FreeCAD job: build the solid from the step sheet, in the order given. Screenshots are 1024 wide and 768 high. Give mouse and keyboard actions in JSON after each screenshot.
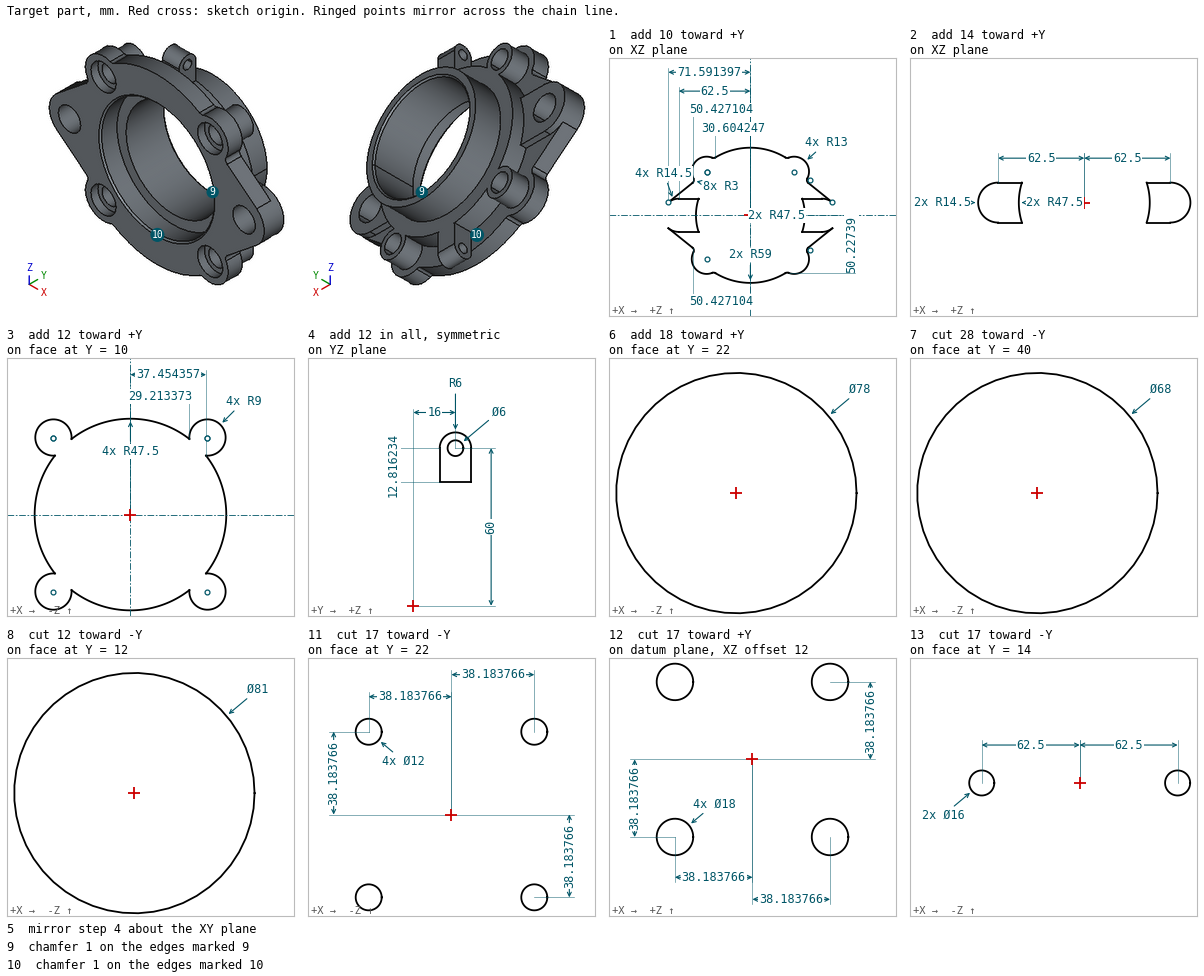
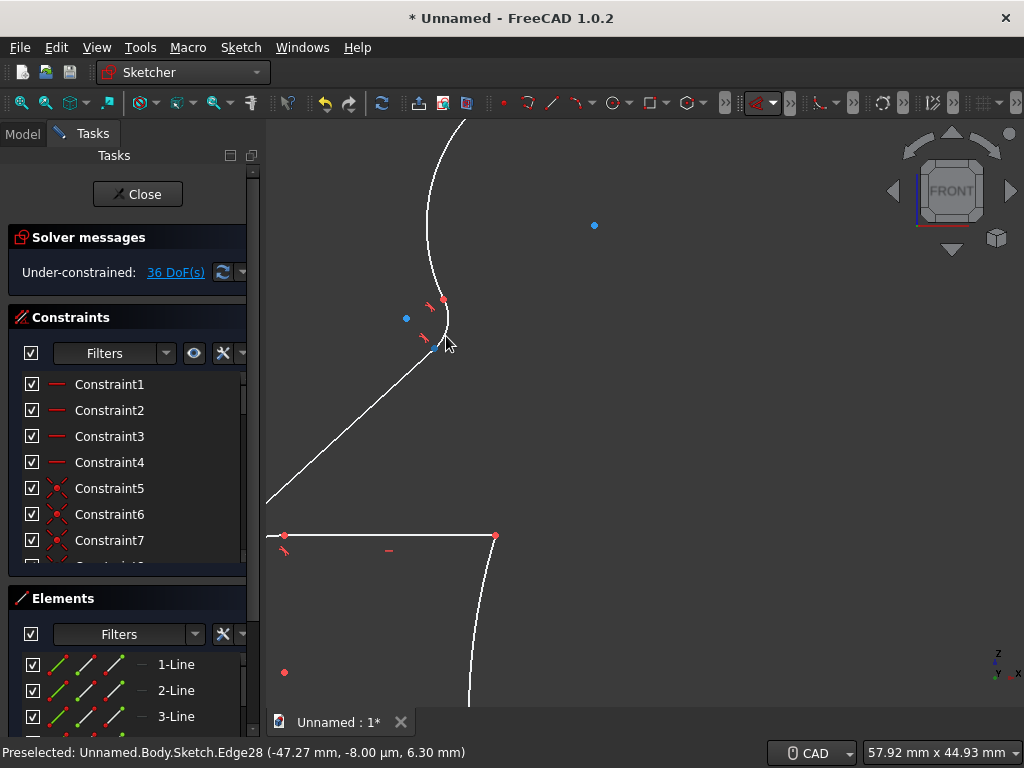
{"action": "left_click", "coordinate": [444, 336]}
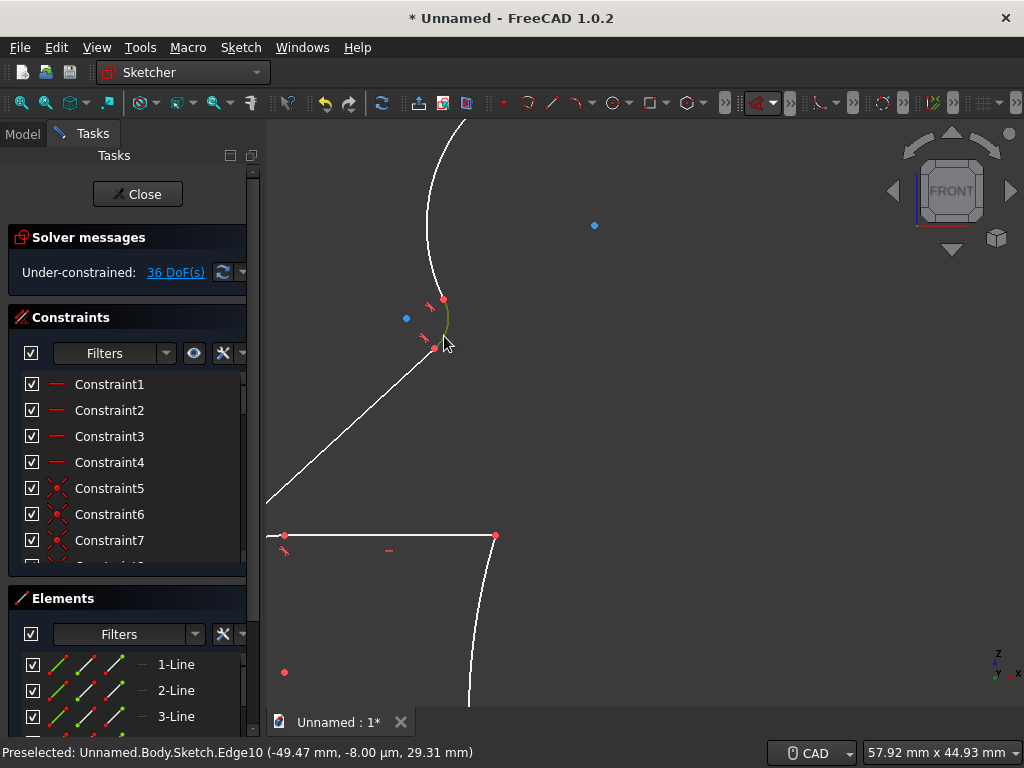
{"action": "scroll", "coordinate": [446, 336], "scroll_direction": "down", "scroll_amount": 8}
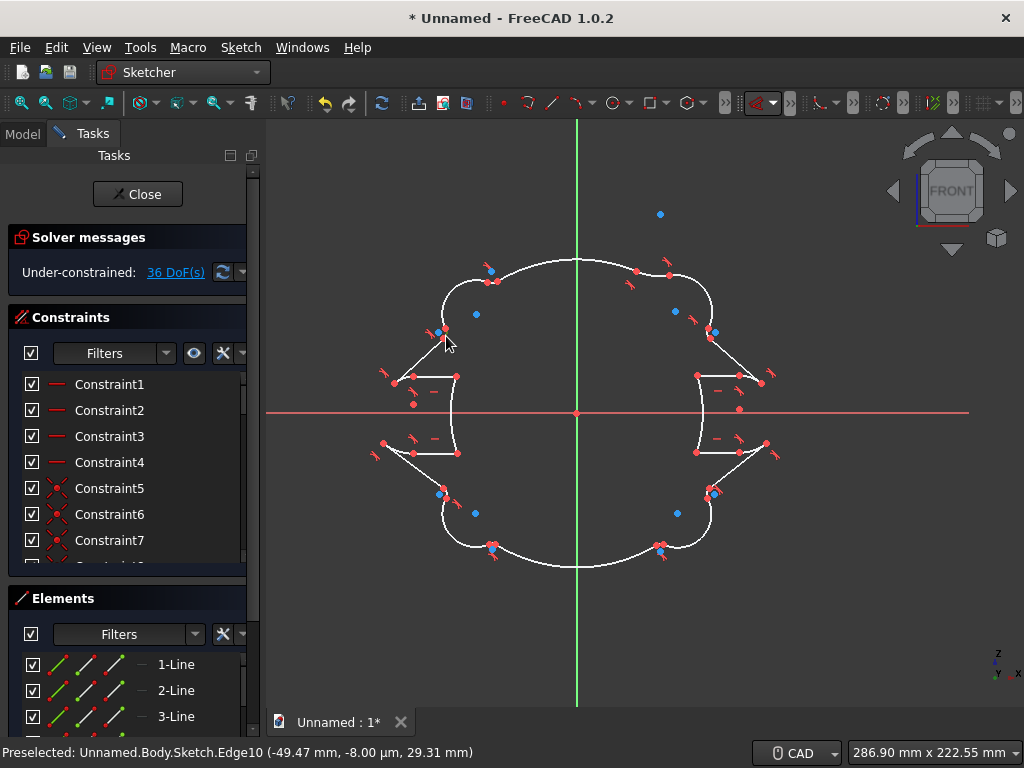
{"action": "scroll", "coordinate": [491, 283], "scroll_direction": "up", "scroll_amount": 8}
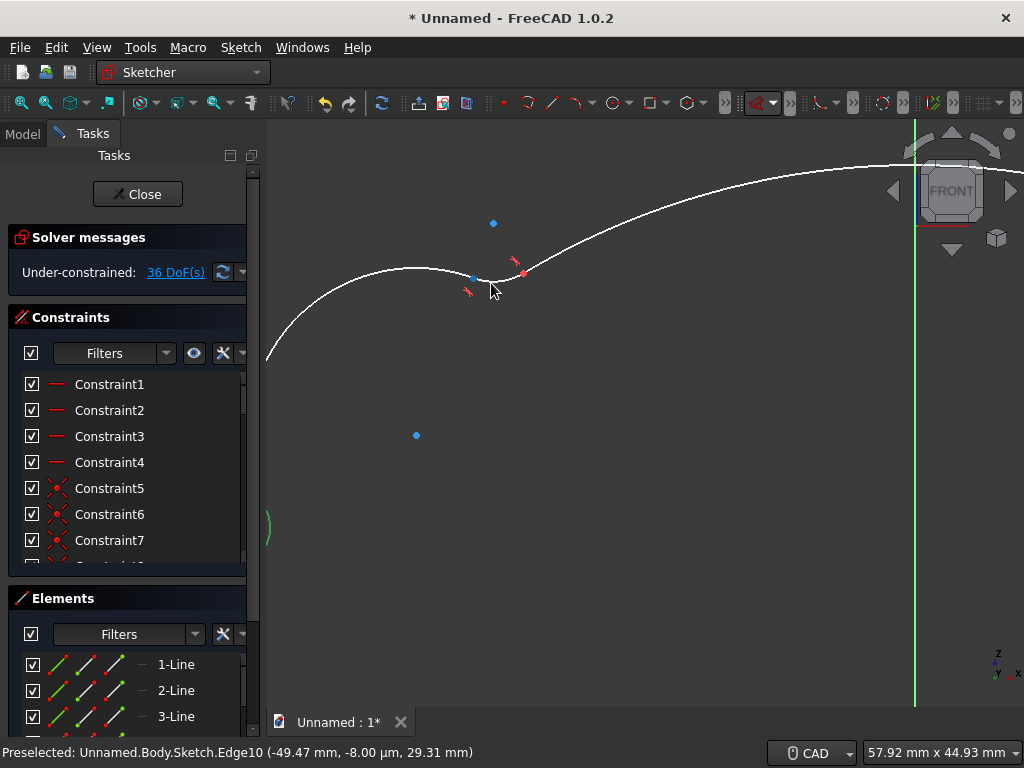
{"action": "left_click", "coordinate": [489, 281]}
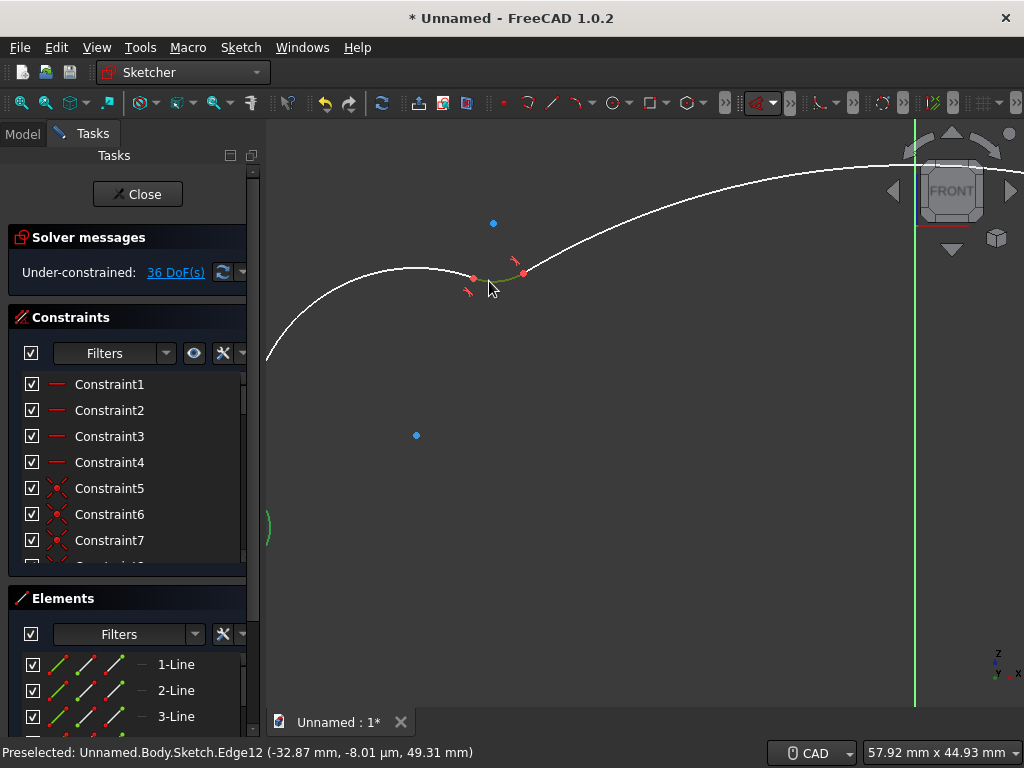
{"action": "scroll", "coordinate": [491, 283], "scroll_direction": "down", "scroll_amount": 8}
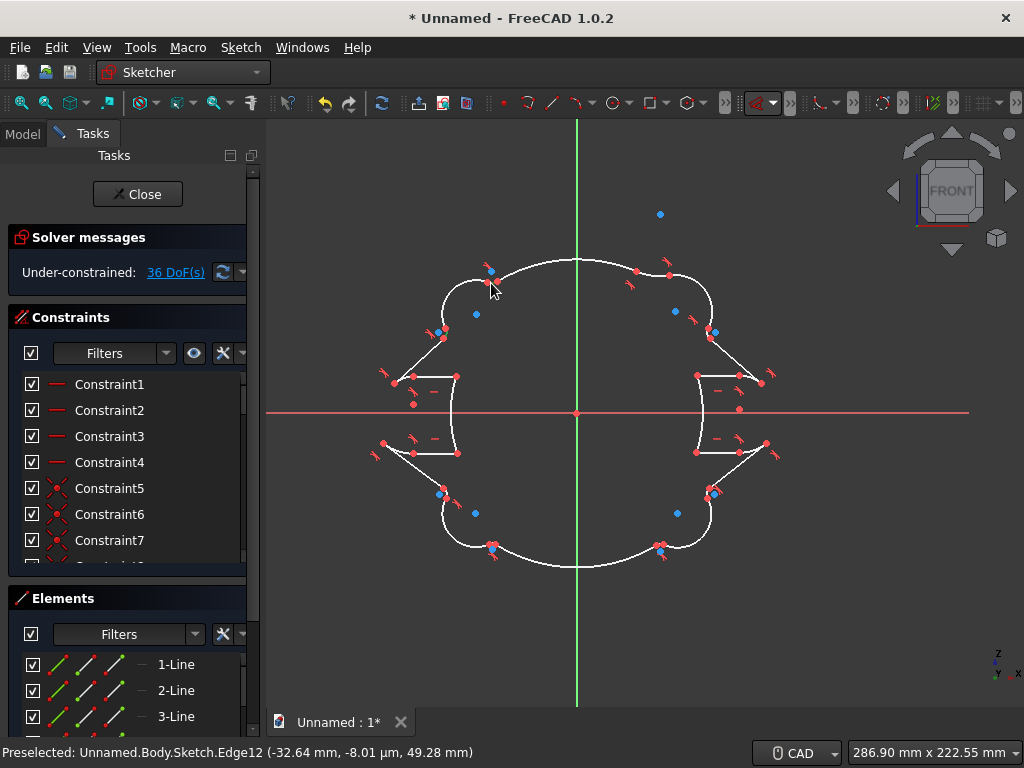
{"action": "scroll", "coordinate": [646, 275], "scroll_direction": "up", "scroll_amount": 2}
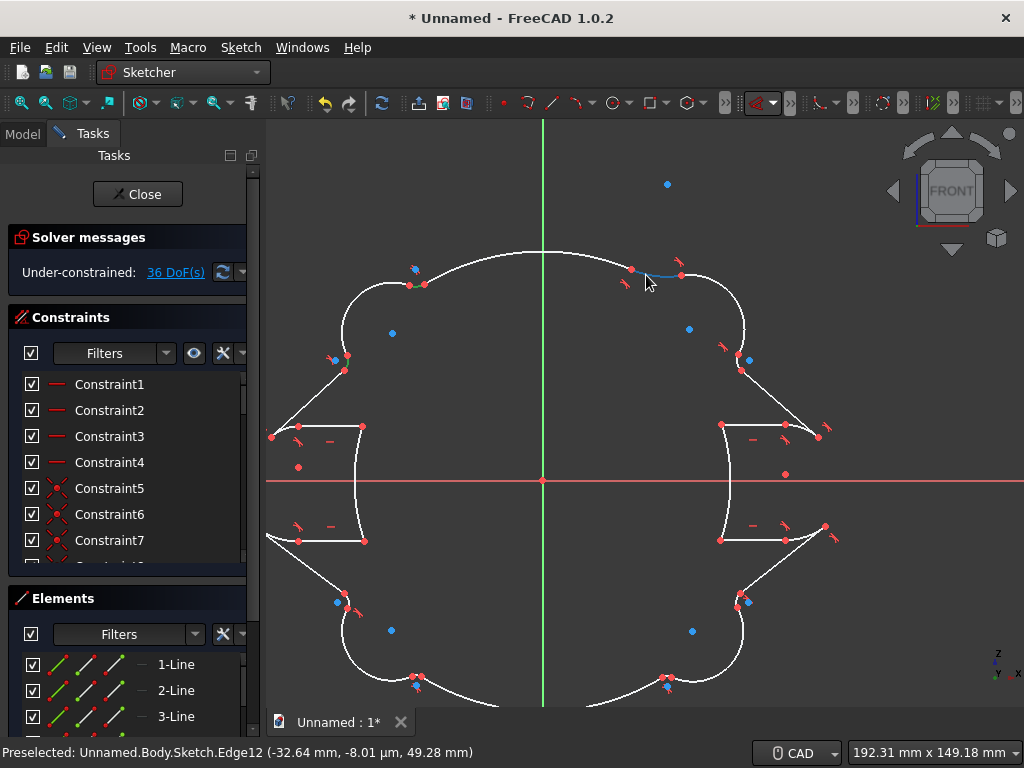
{"action": "left_click", "coordinate": [646, 274]}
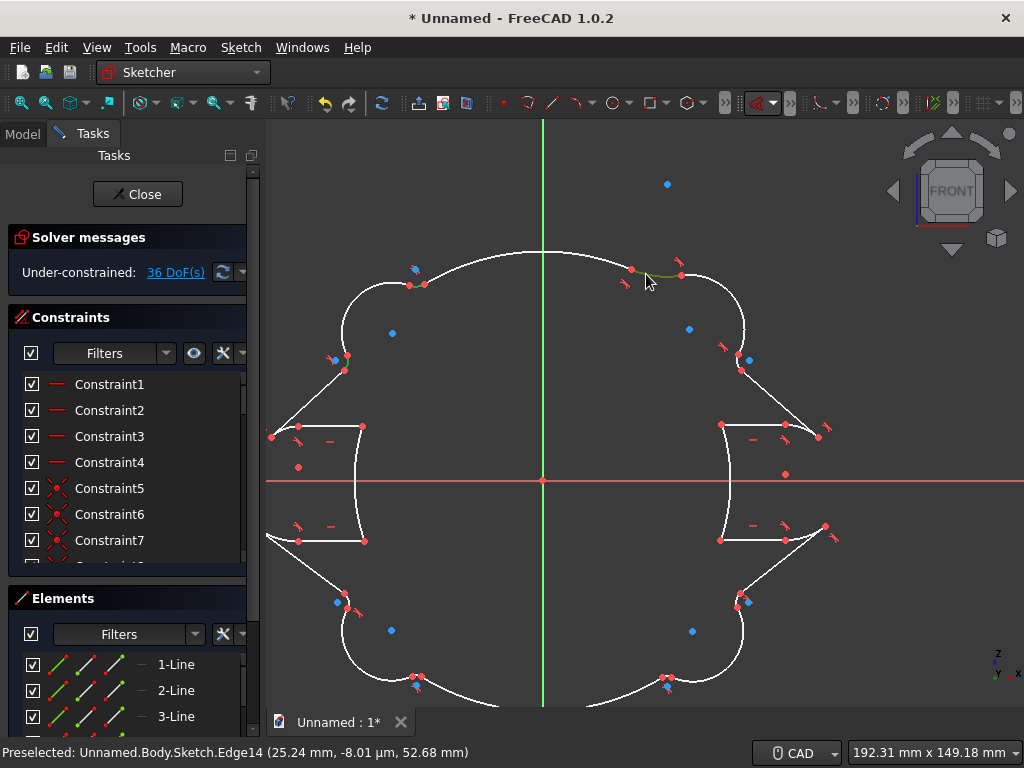
{"action": "scroll", "coordinate": [737, 363], "scroll_direction": "up", "scroll_amount": 3}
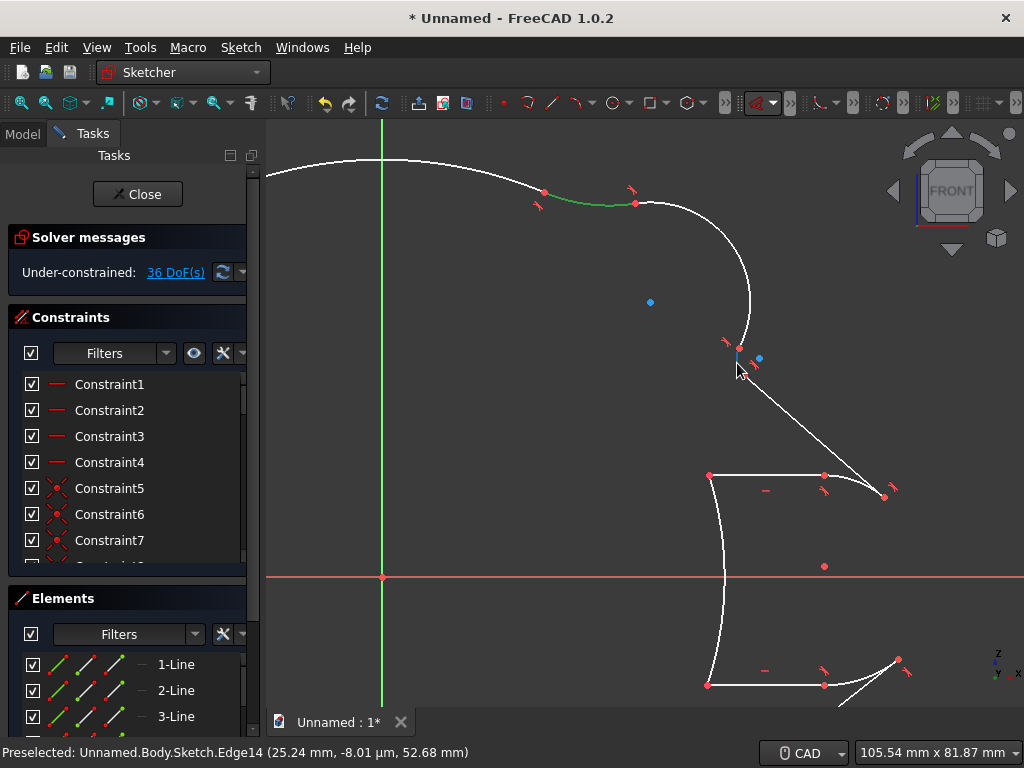
{"action": "left_click", "coordinate": [737, 363]}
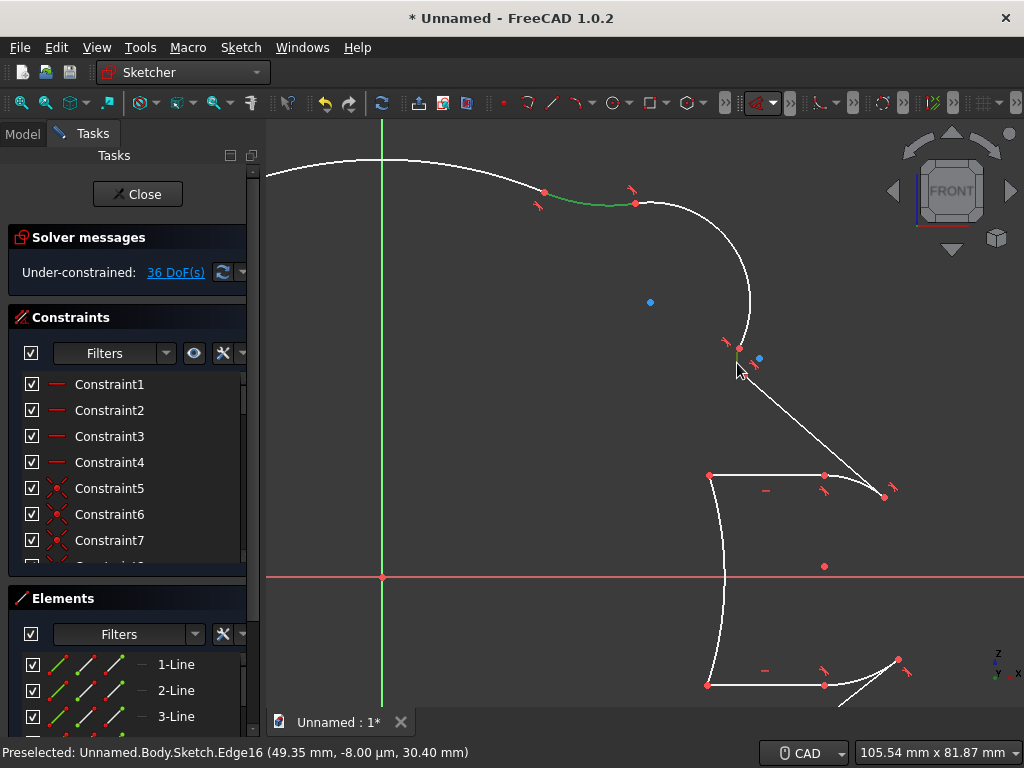
{"action": "scroll", "coordinate": [690, 317], "scroll_direction": "down", "scroll_amount": 5}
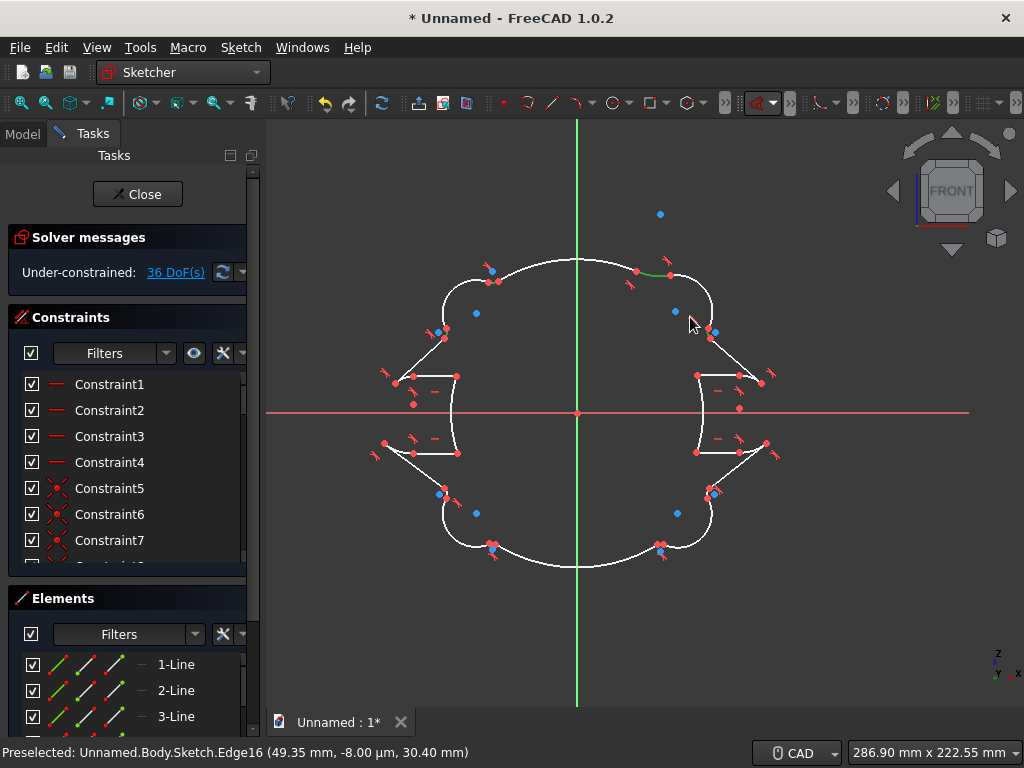
{"action": "scroll", "coordinate": [707, 493], "scroll_direction": "up", "scroll_amount": 5}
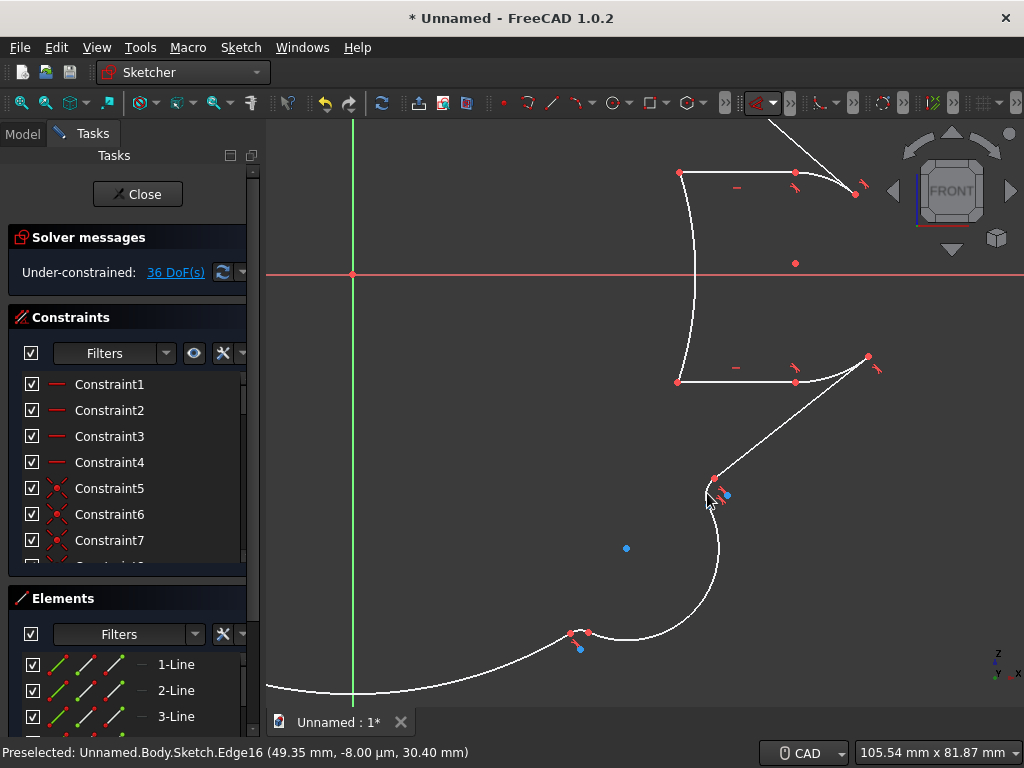
{"action": "left_click", "coordinate": [706, 491]}